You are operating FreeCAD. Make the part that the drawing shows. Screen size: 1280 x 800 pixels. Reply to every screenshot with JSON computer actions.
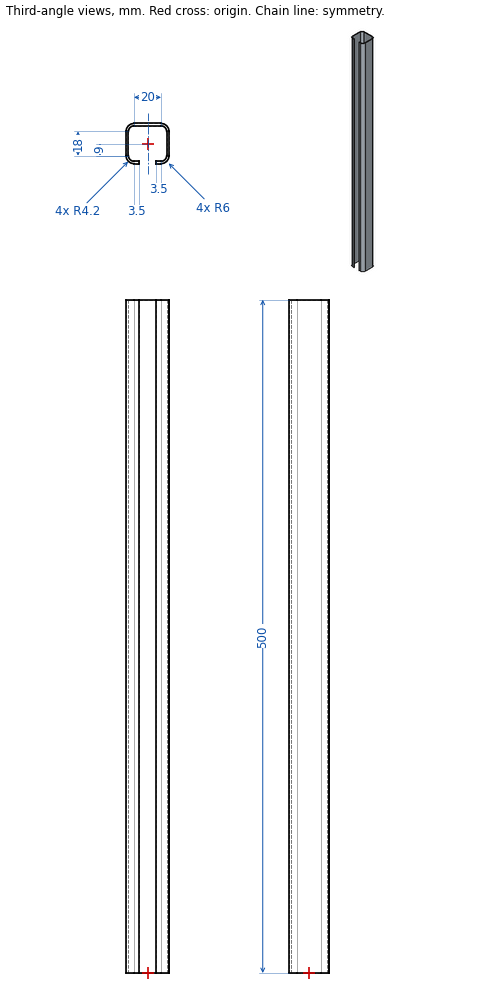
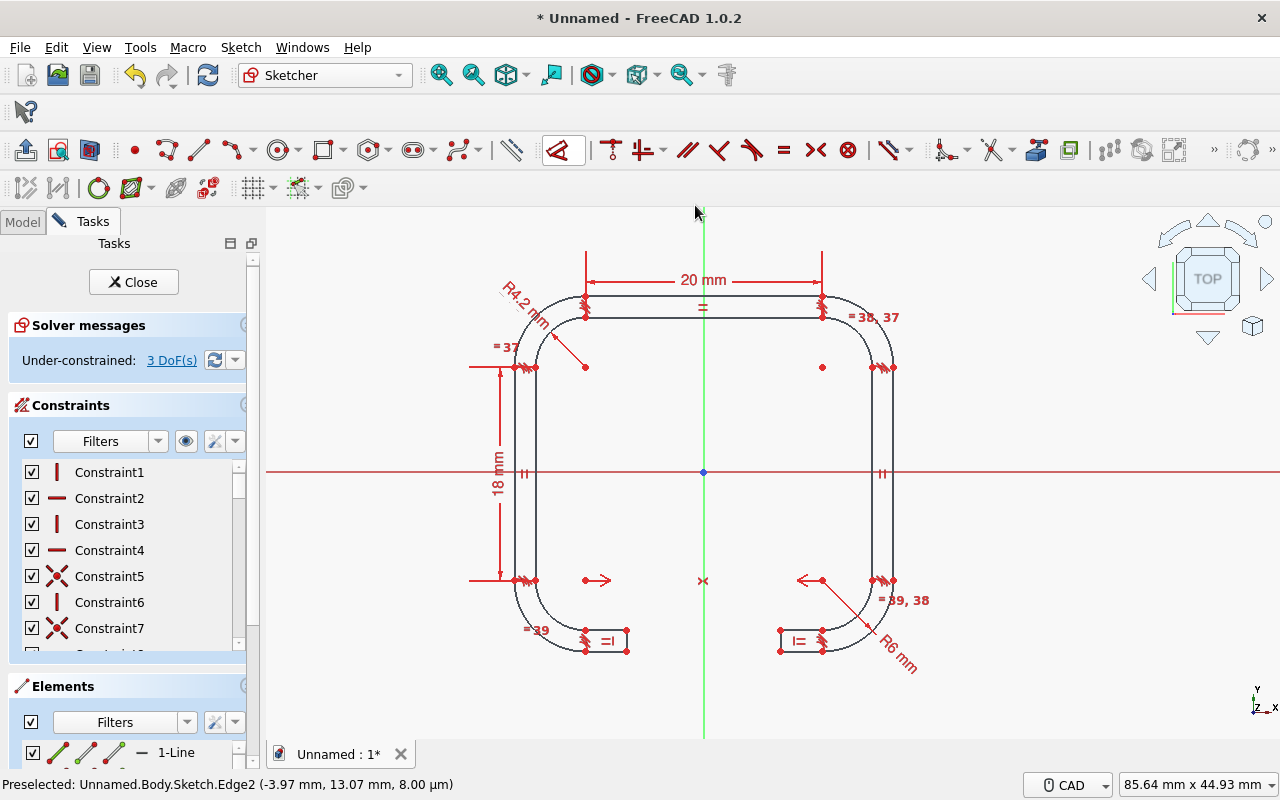
{"action": "left_click", "coordinate": [536, 581]}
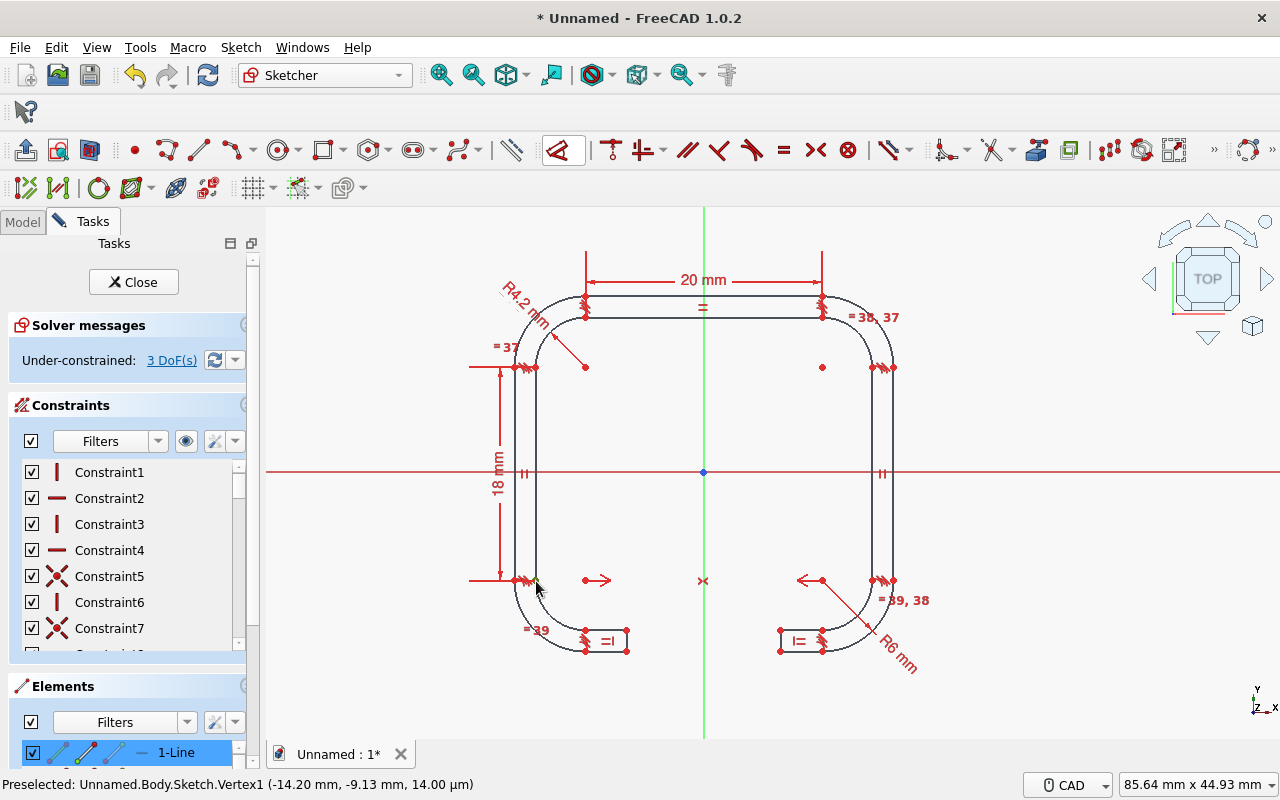
{"action": "key", "text": "i"}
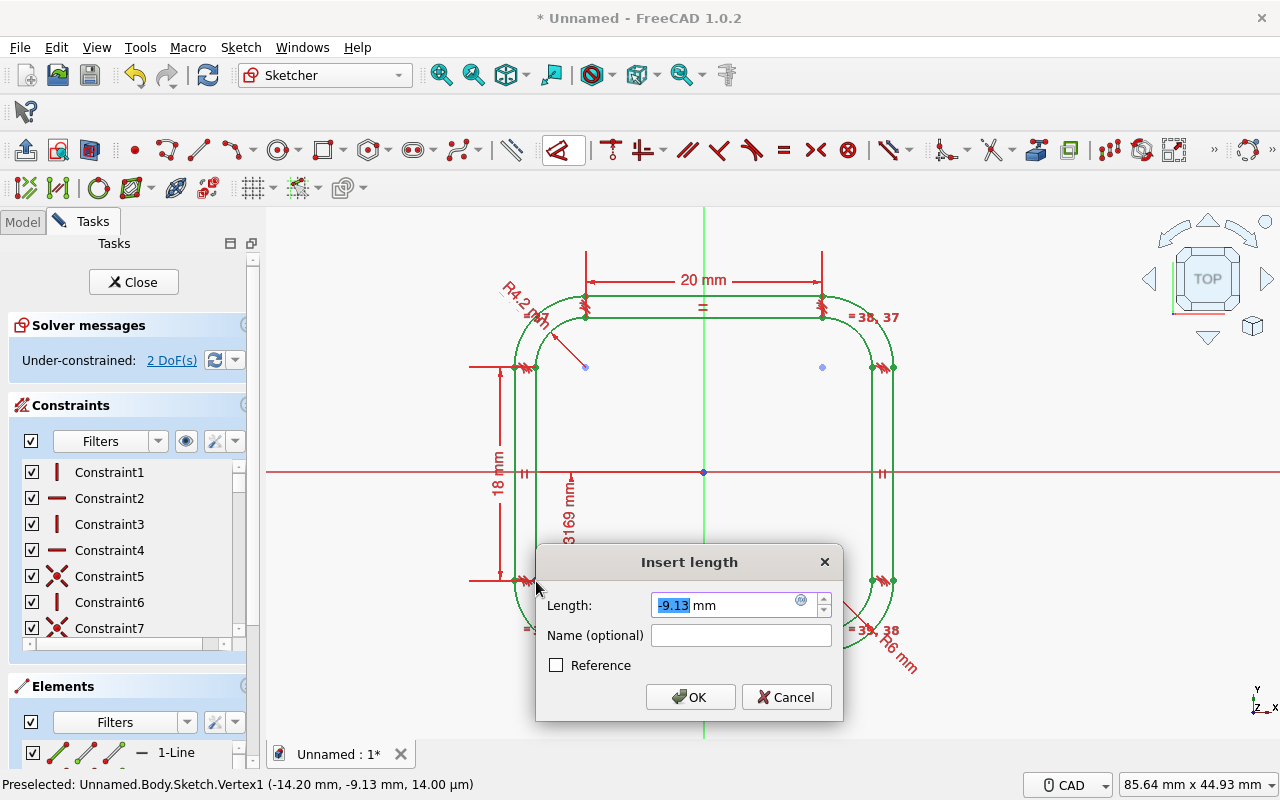
{"action": "type", "text": "-9"}
{"action": "key", "text": "Return"}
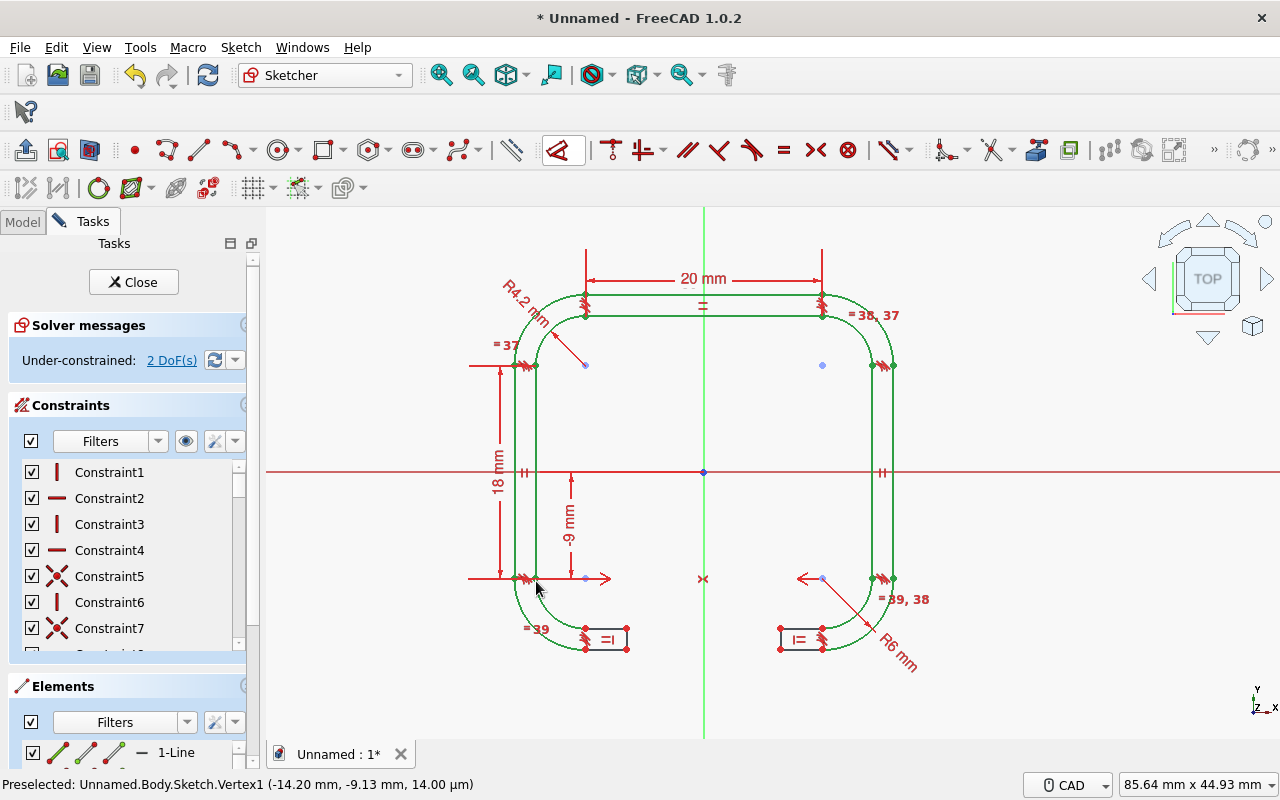
{"action": "left_click", "coordinate": [810, 629]}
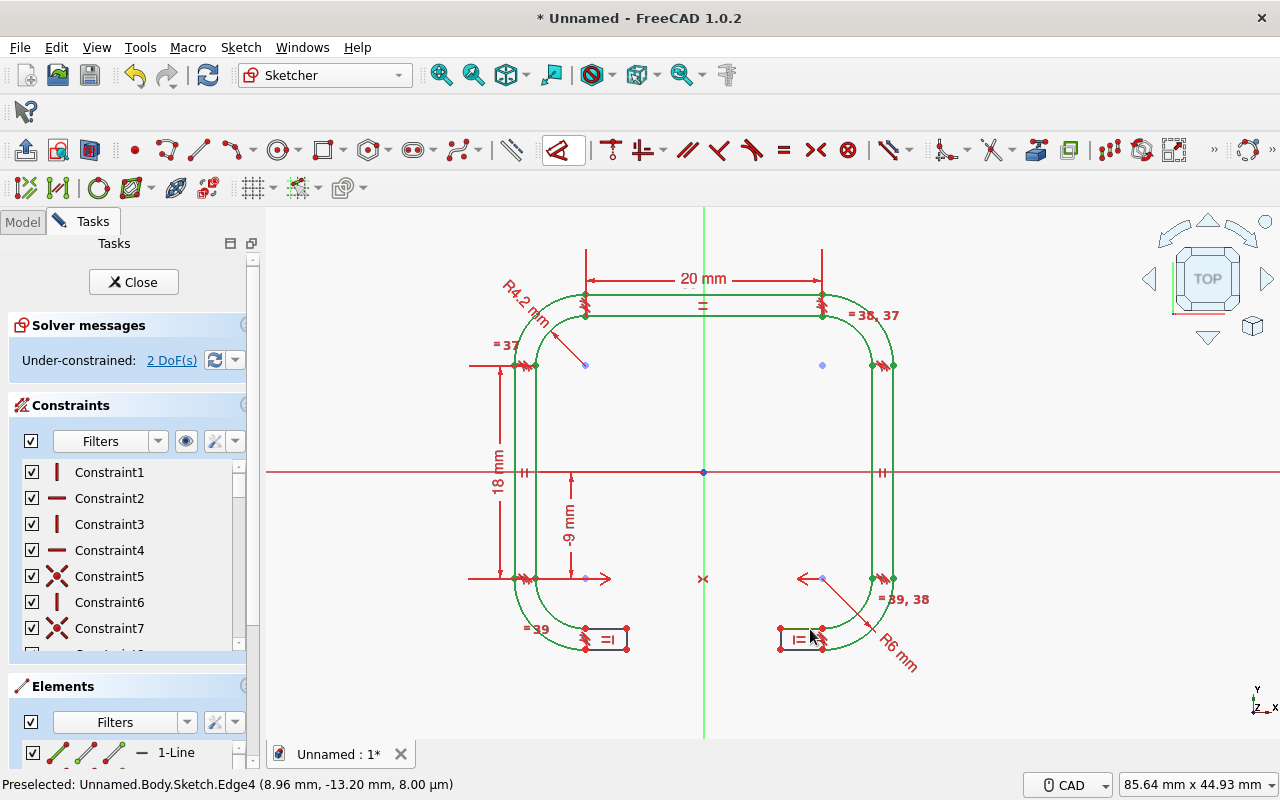
{"action": "left_click", "coordinate": [580, 150]}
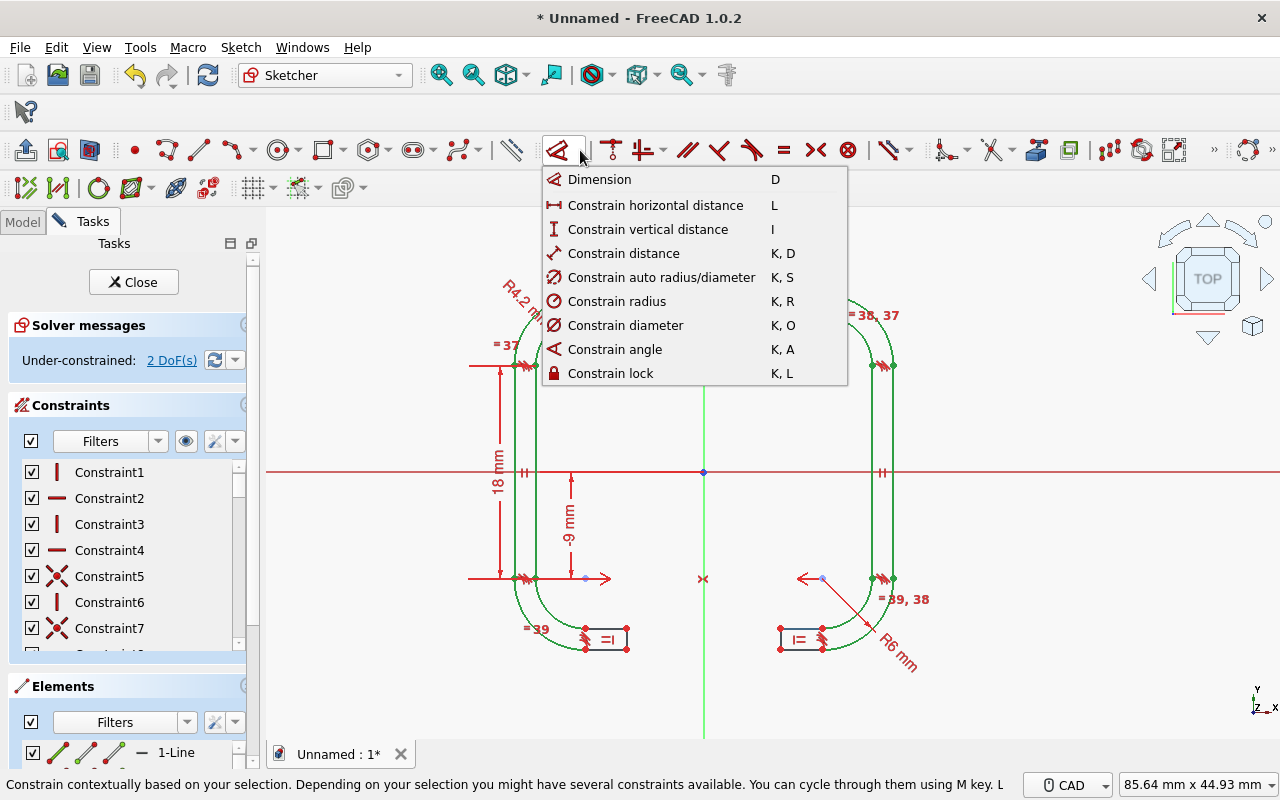
{"action": "left_click", "coordinate": [695, 205]}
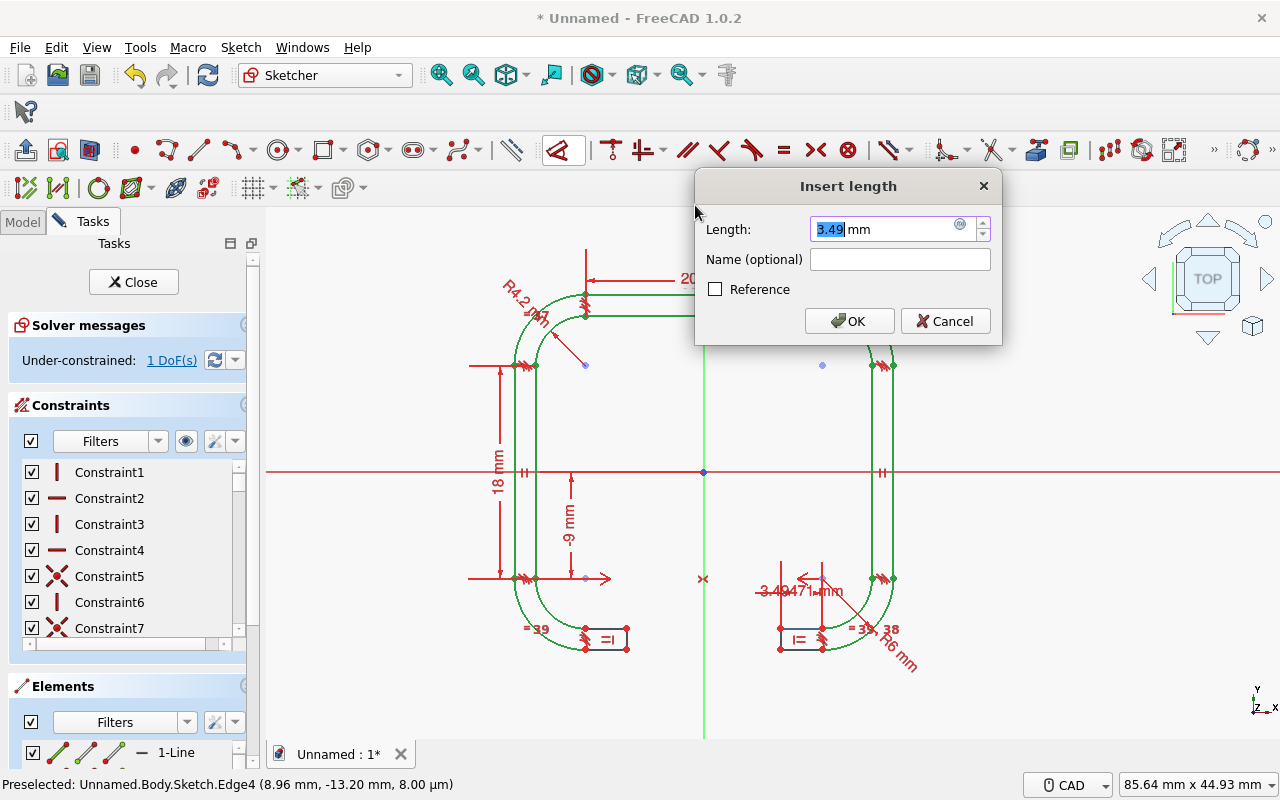
{"action": "type", "text": "3.5"}
{"action": "key", "text": "Return"}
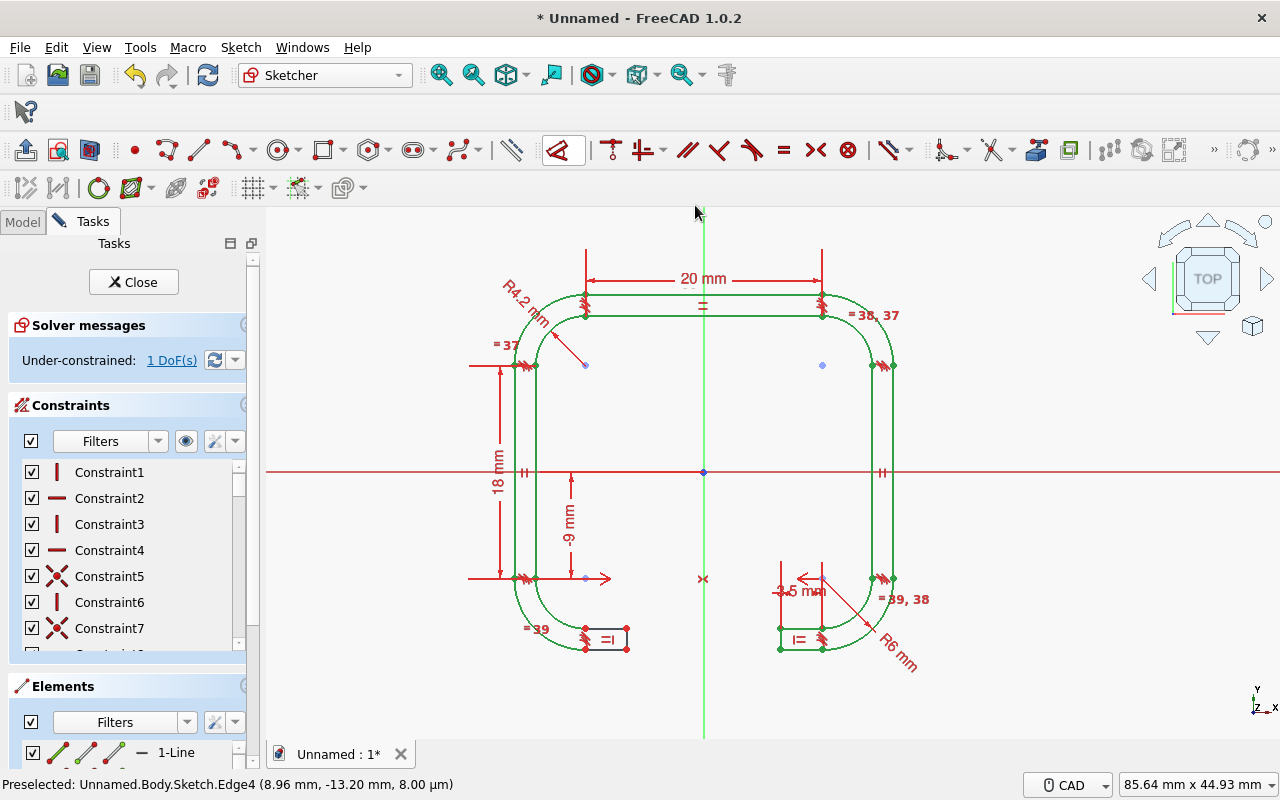
{"action": "left_click", "coordinate": [598, 650]}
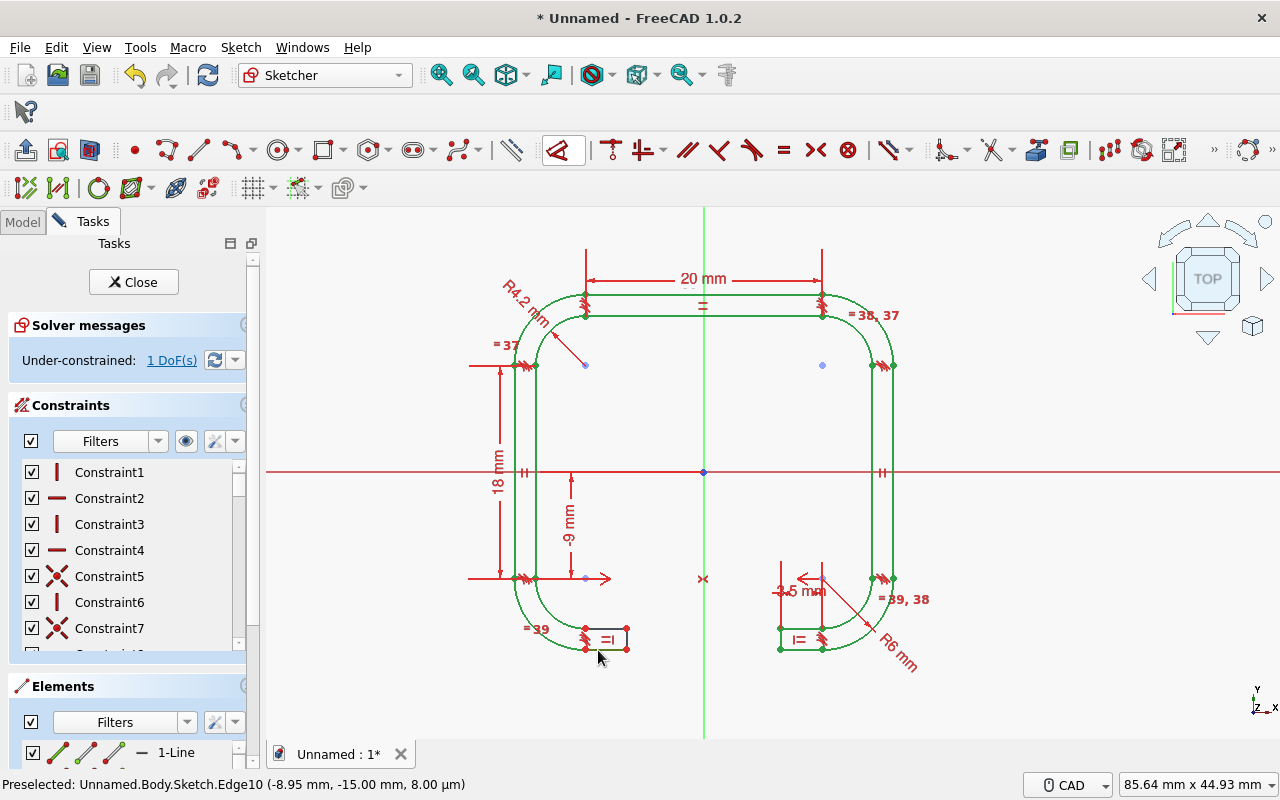
{"action": "left_click", "coordinate": [580, 150]}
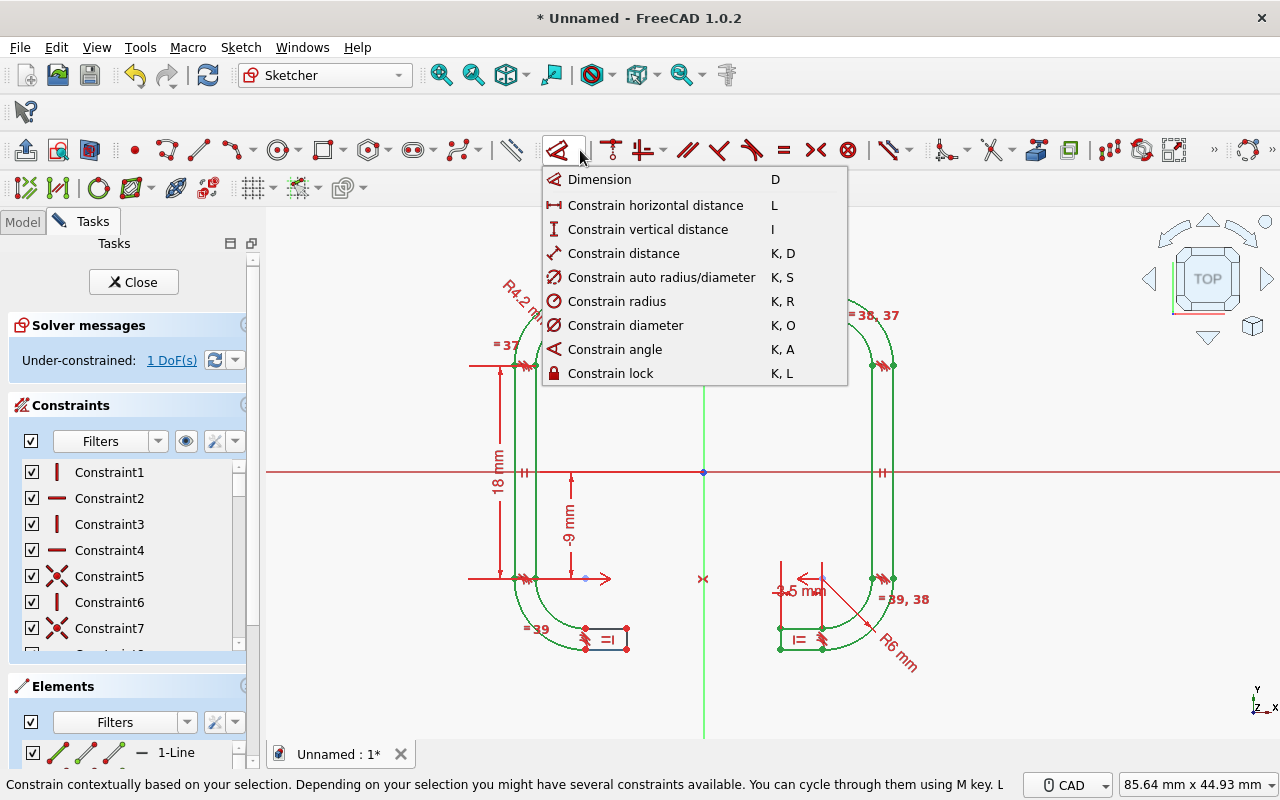
{"action": "left_click", "coordinate": [695, 205]}